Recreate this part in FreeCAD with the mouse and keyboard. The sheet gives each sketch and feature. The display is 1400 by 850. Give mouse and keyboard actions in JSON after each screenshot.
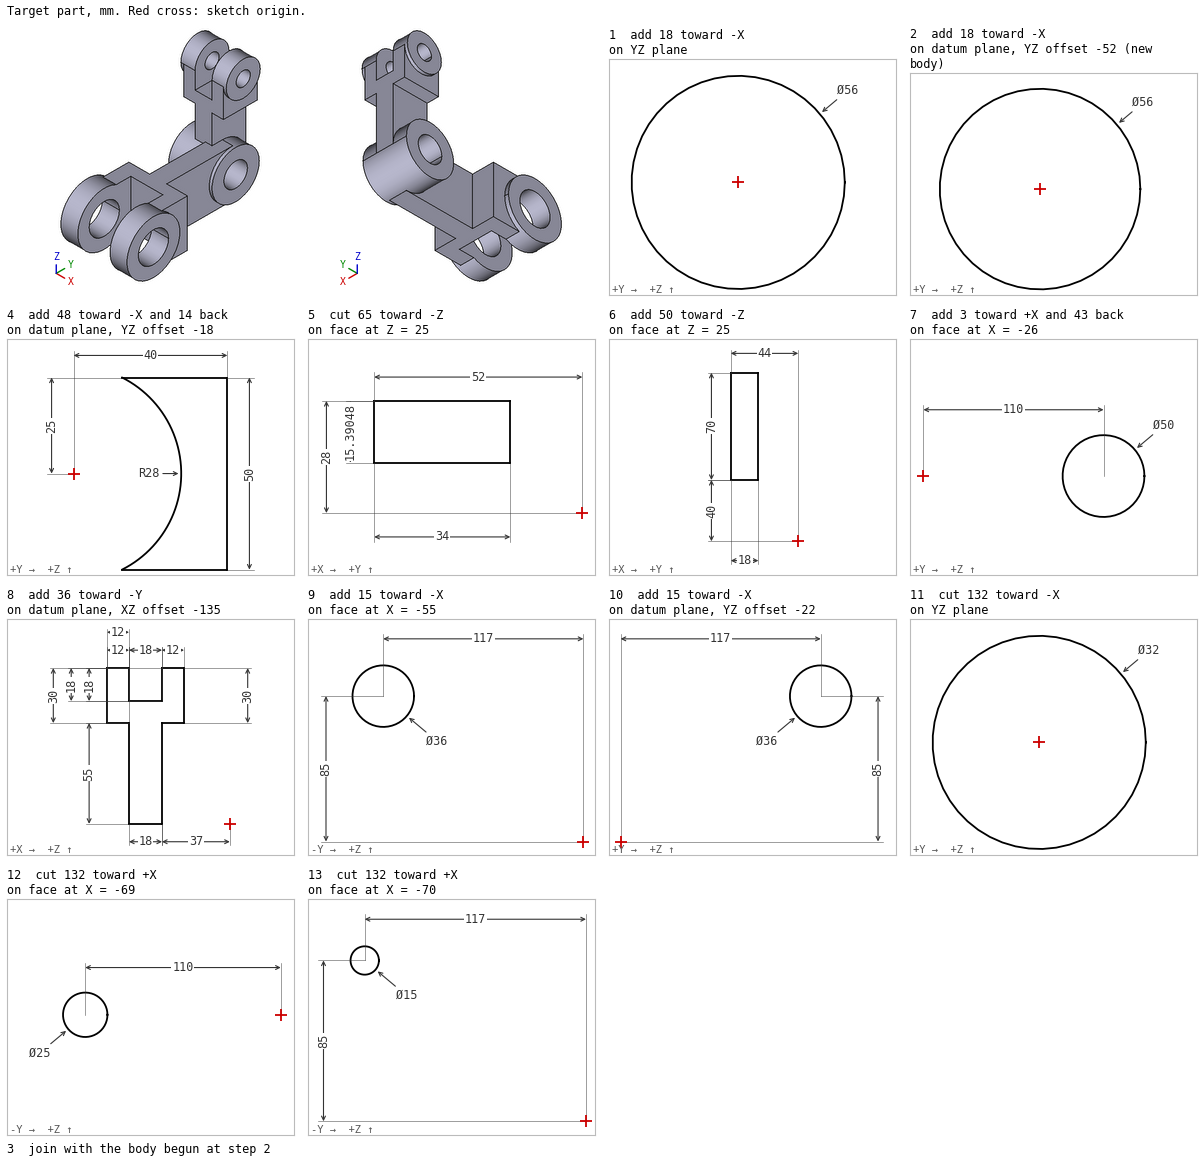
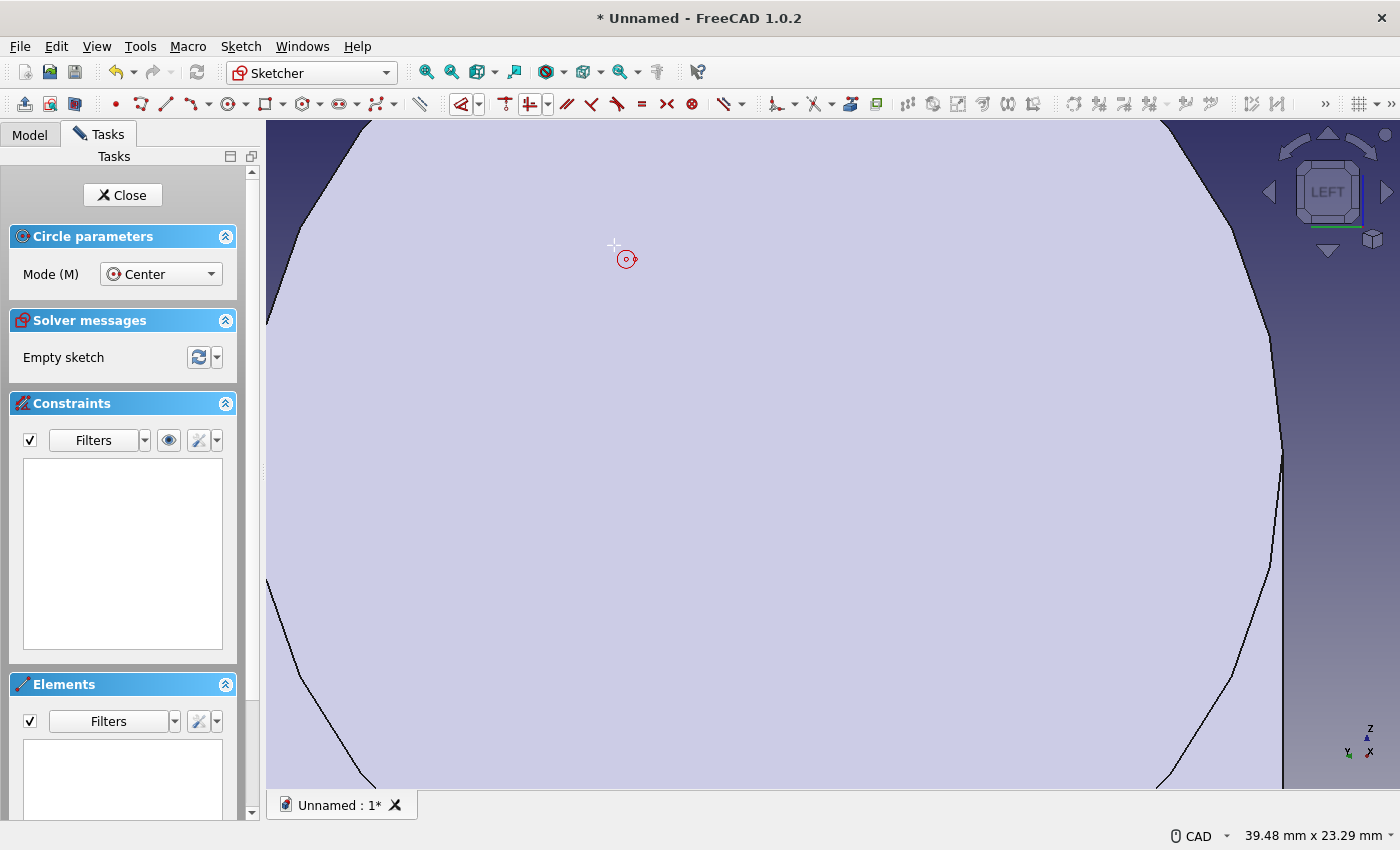
{"action": "left_click", "coordinate": [766, 452]}
{"action": "left_click", "coordinate": [918, 300]}
{"action": "key", "text": "Escape"}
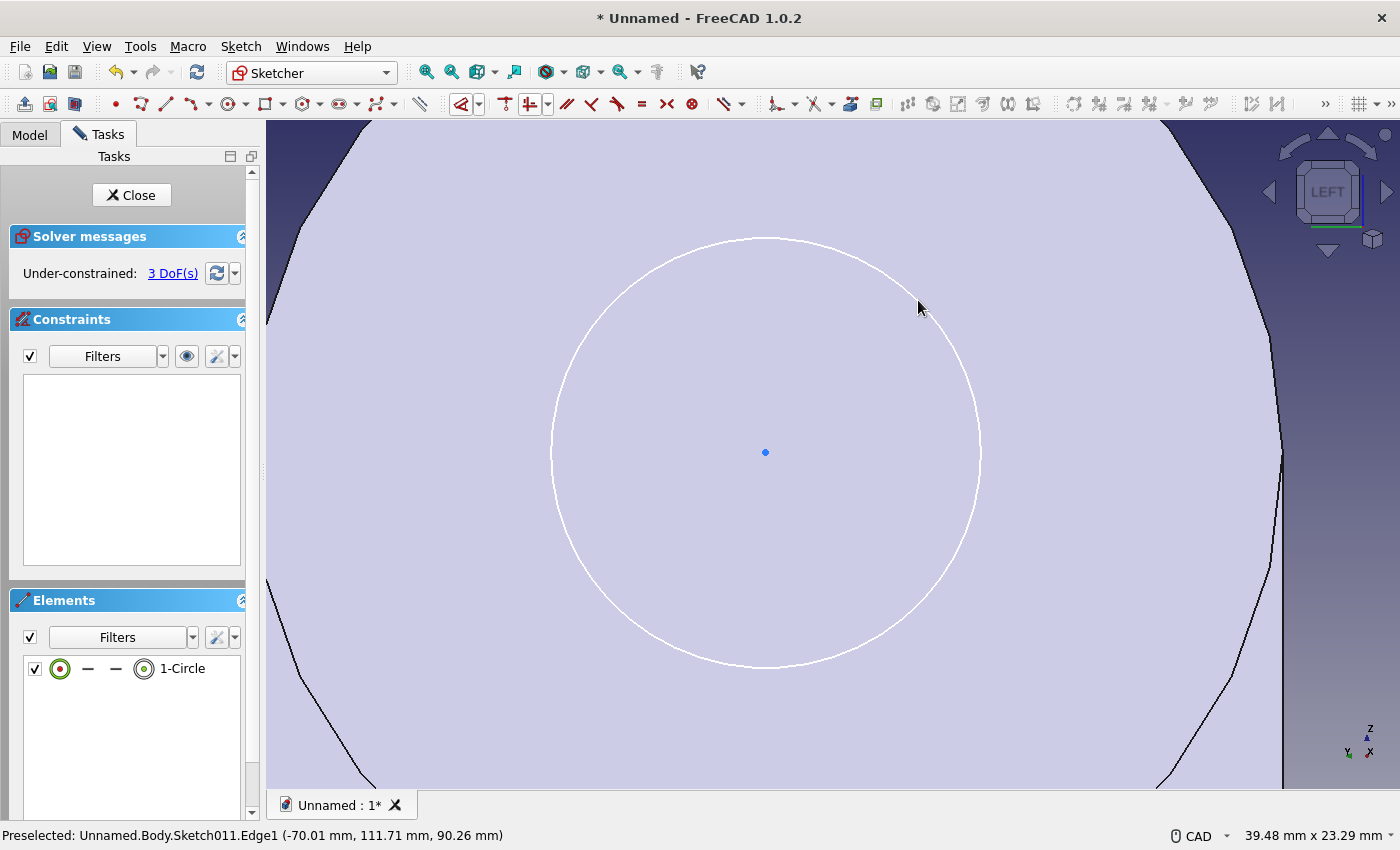
{"action": "left_click", "coordinate": [918, 301]}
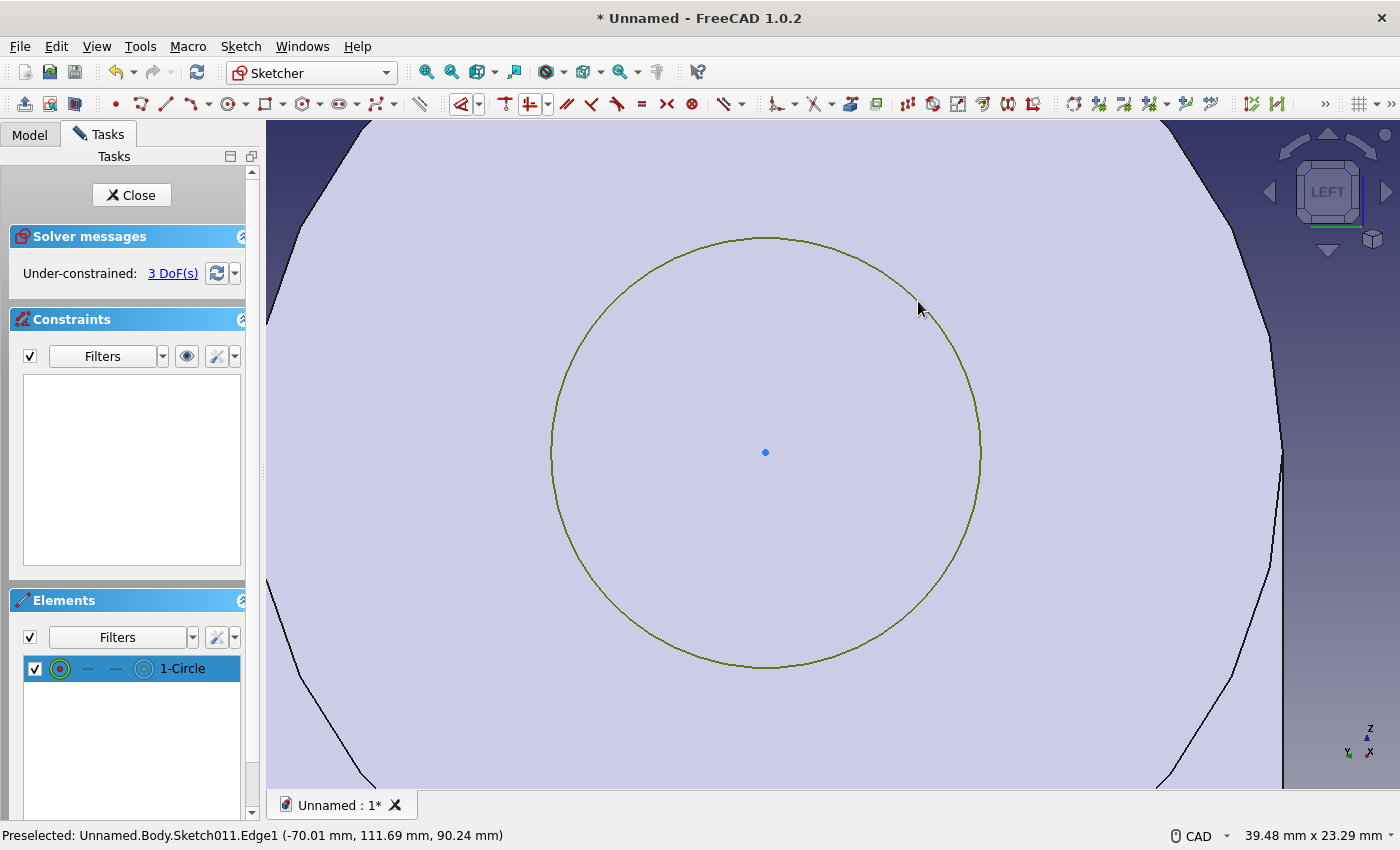
{"action": "key", "text": "k o"}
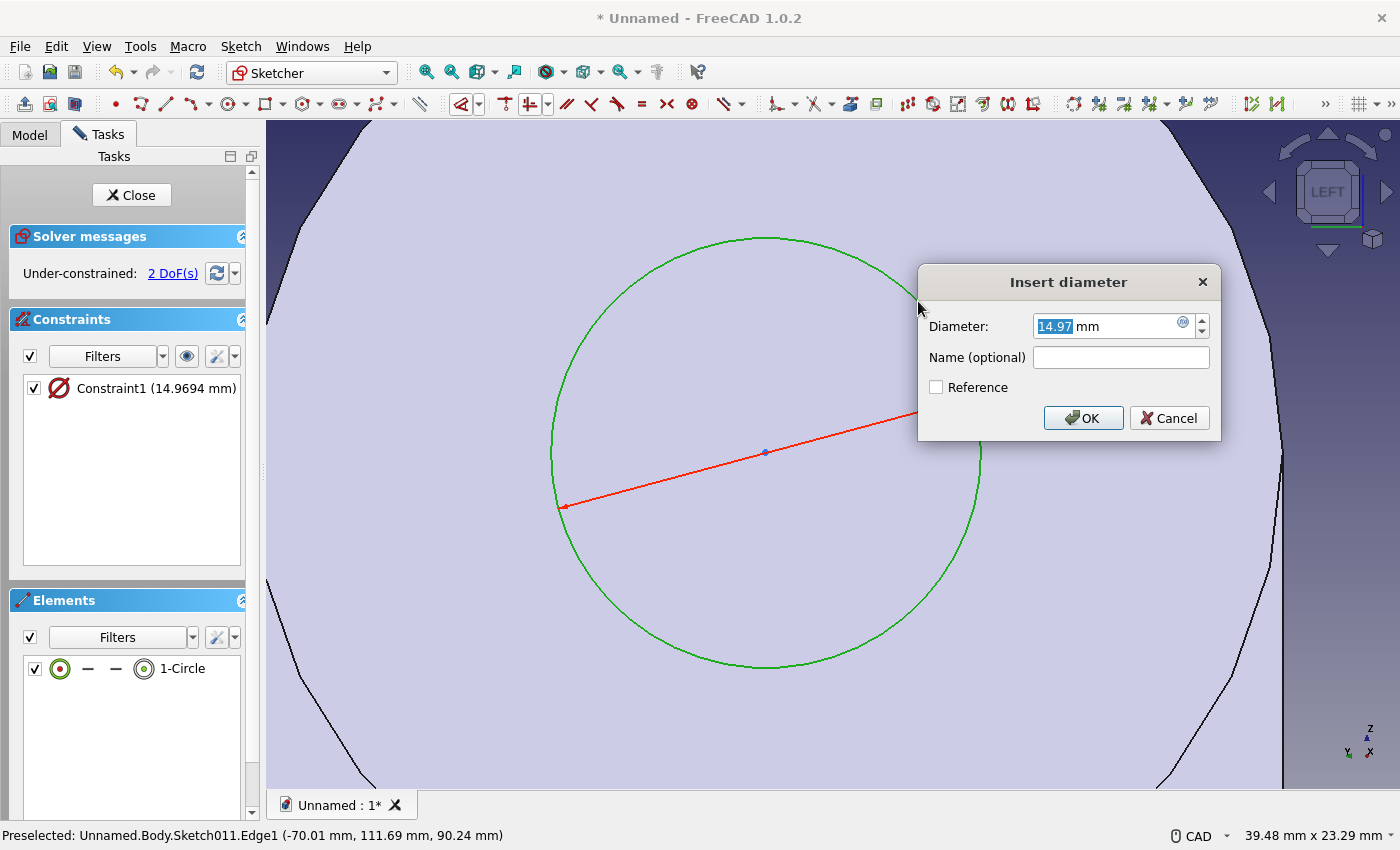
{"action": "type", "text": "15"}
{"action": "key", "text": "Return"}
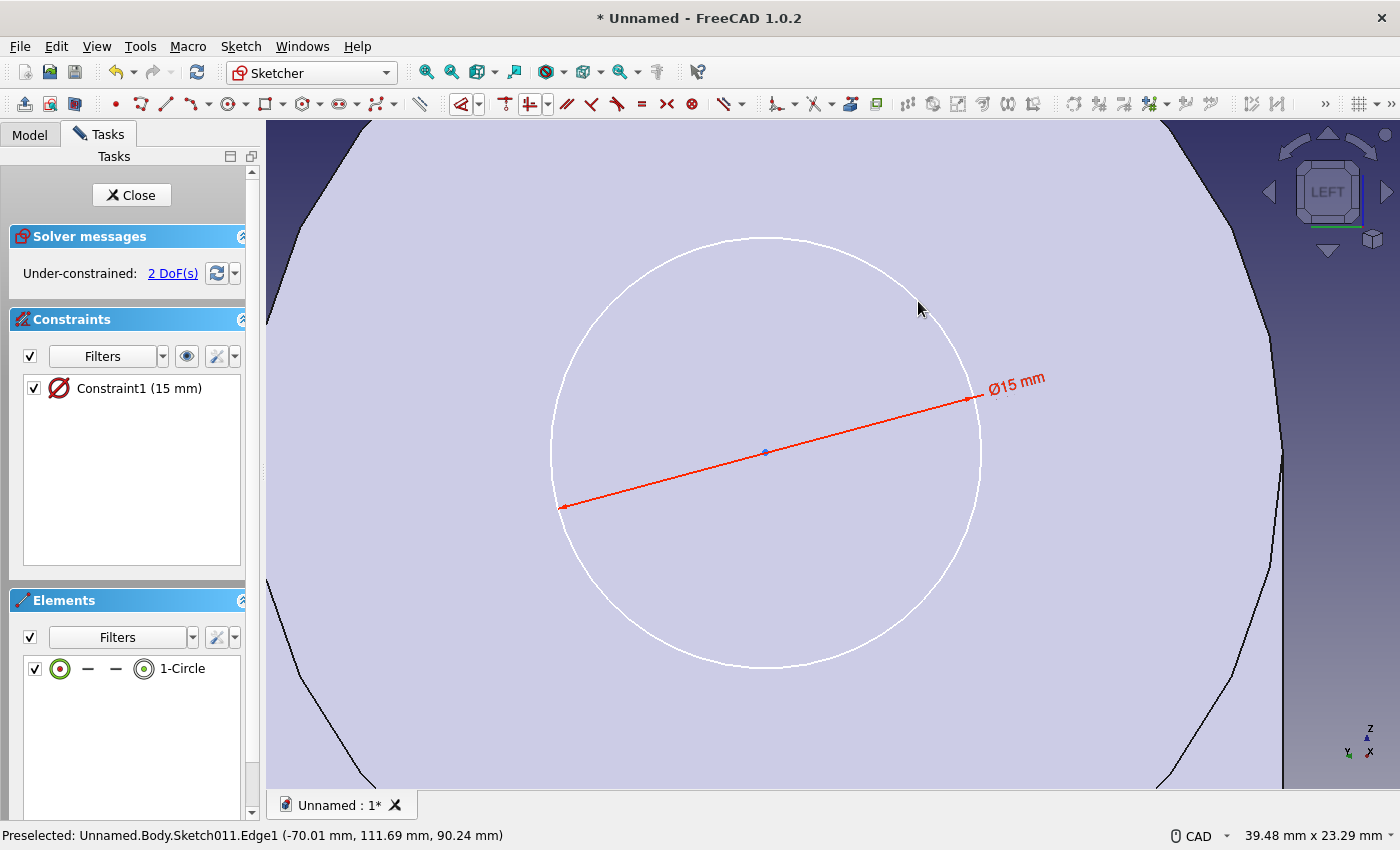
{"action": "left_click", "coordinate": [766, 453]}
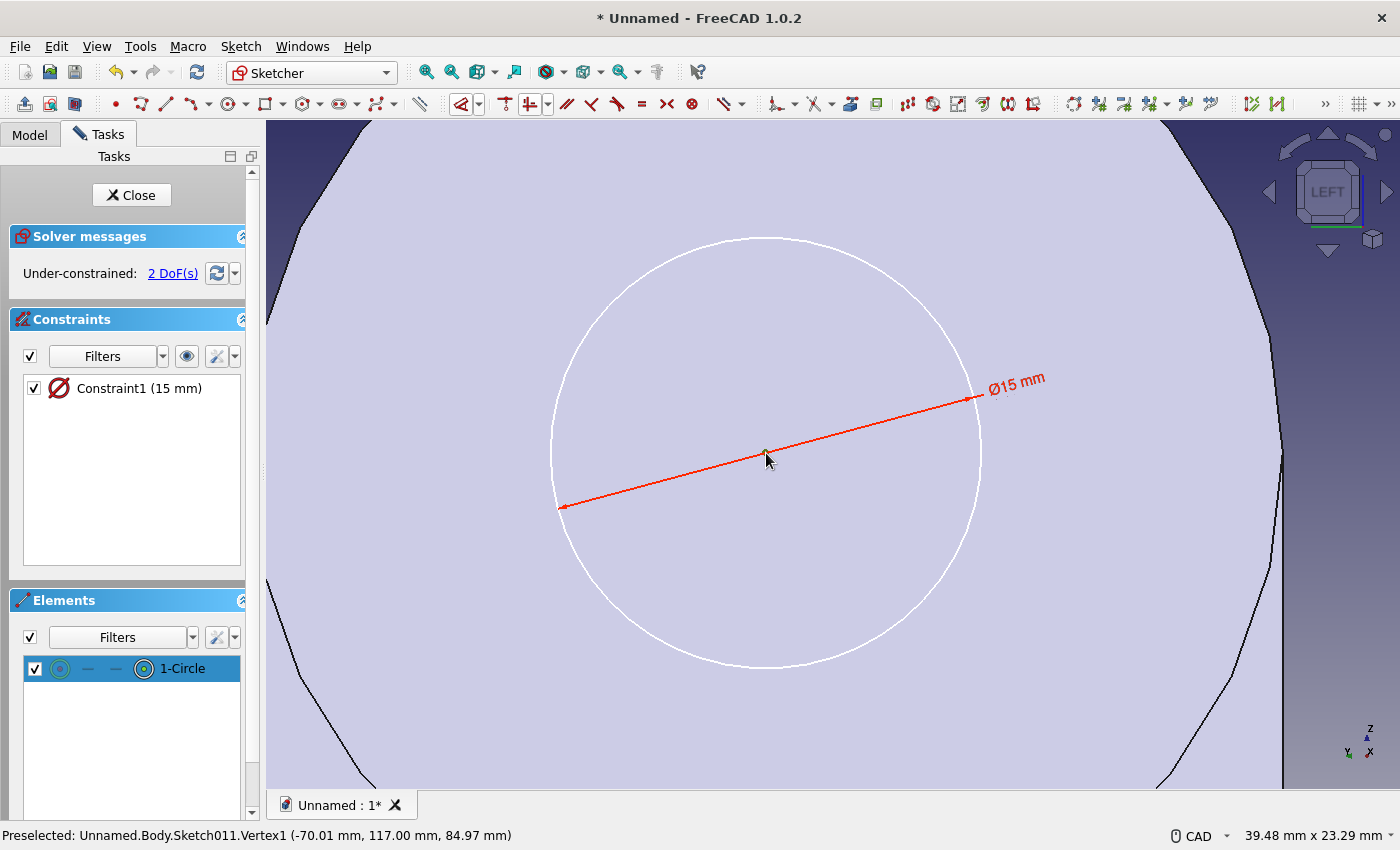
{"action": "key", "text": "i"}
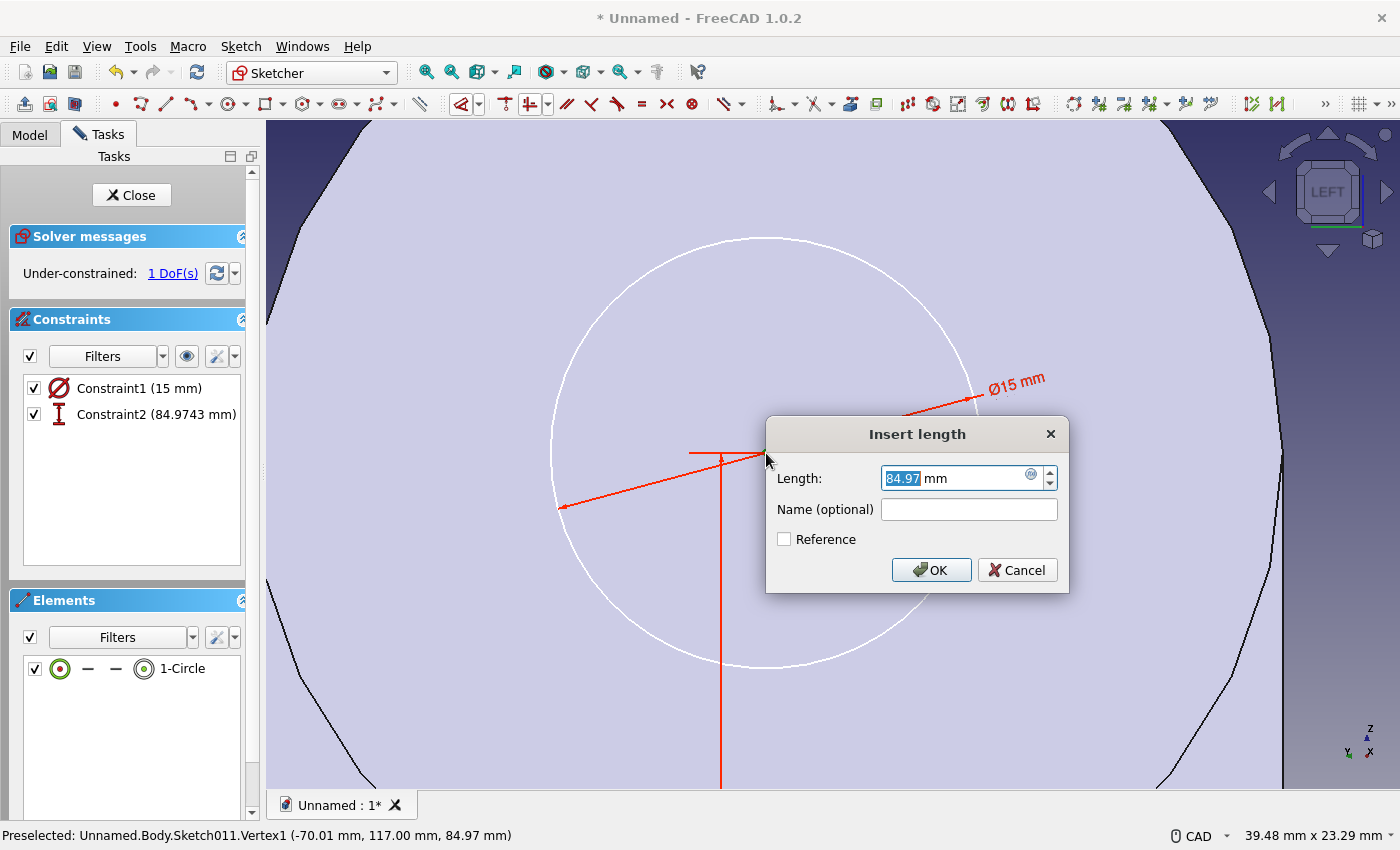
{"action": "type", "text": "85"}
{"action": "key", "text": "Return"}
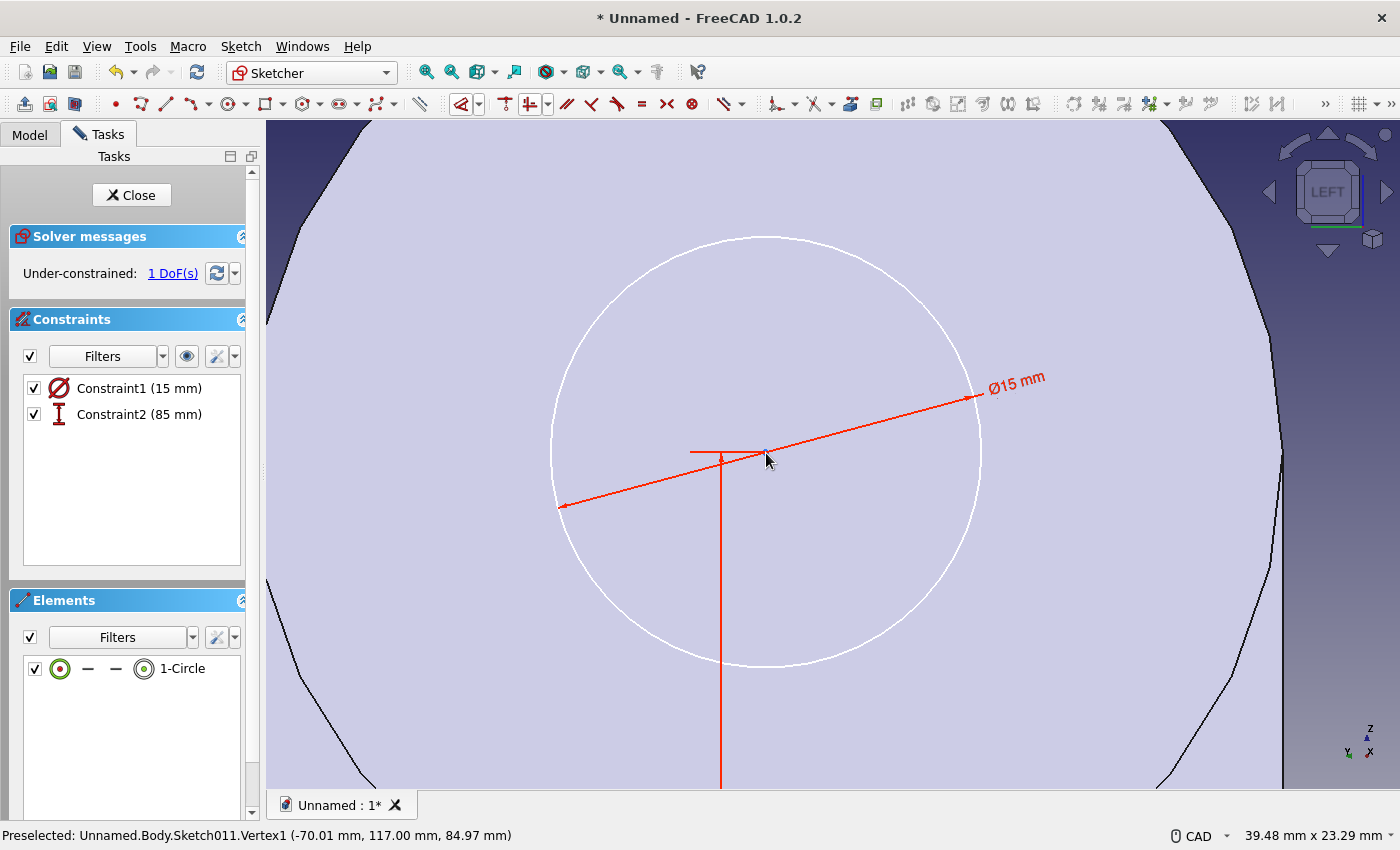
{"action": "left_click", "coordinate": [766, 452]}